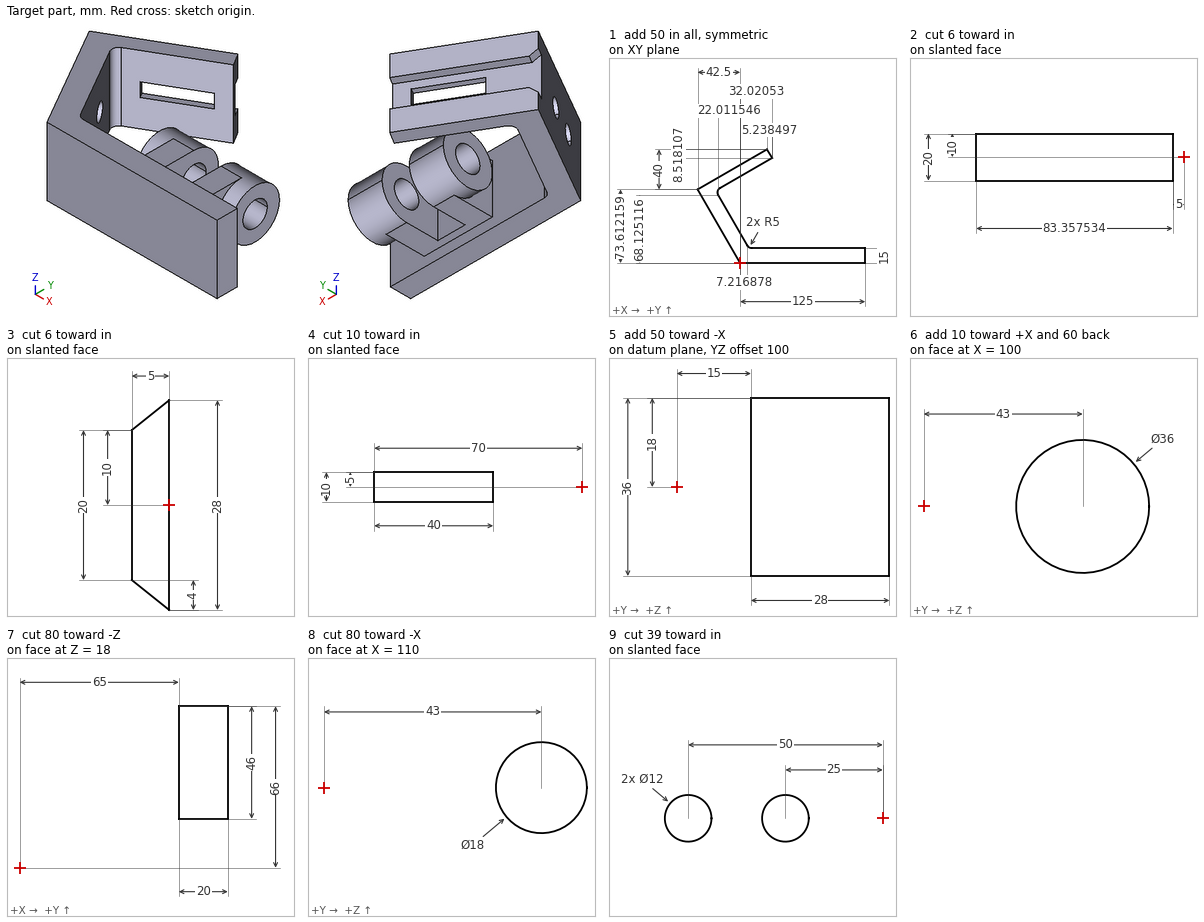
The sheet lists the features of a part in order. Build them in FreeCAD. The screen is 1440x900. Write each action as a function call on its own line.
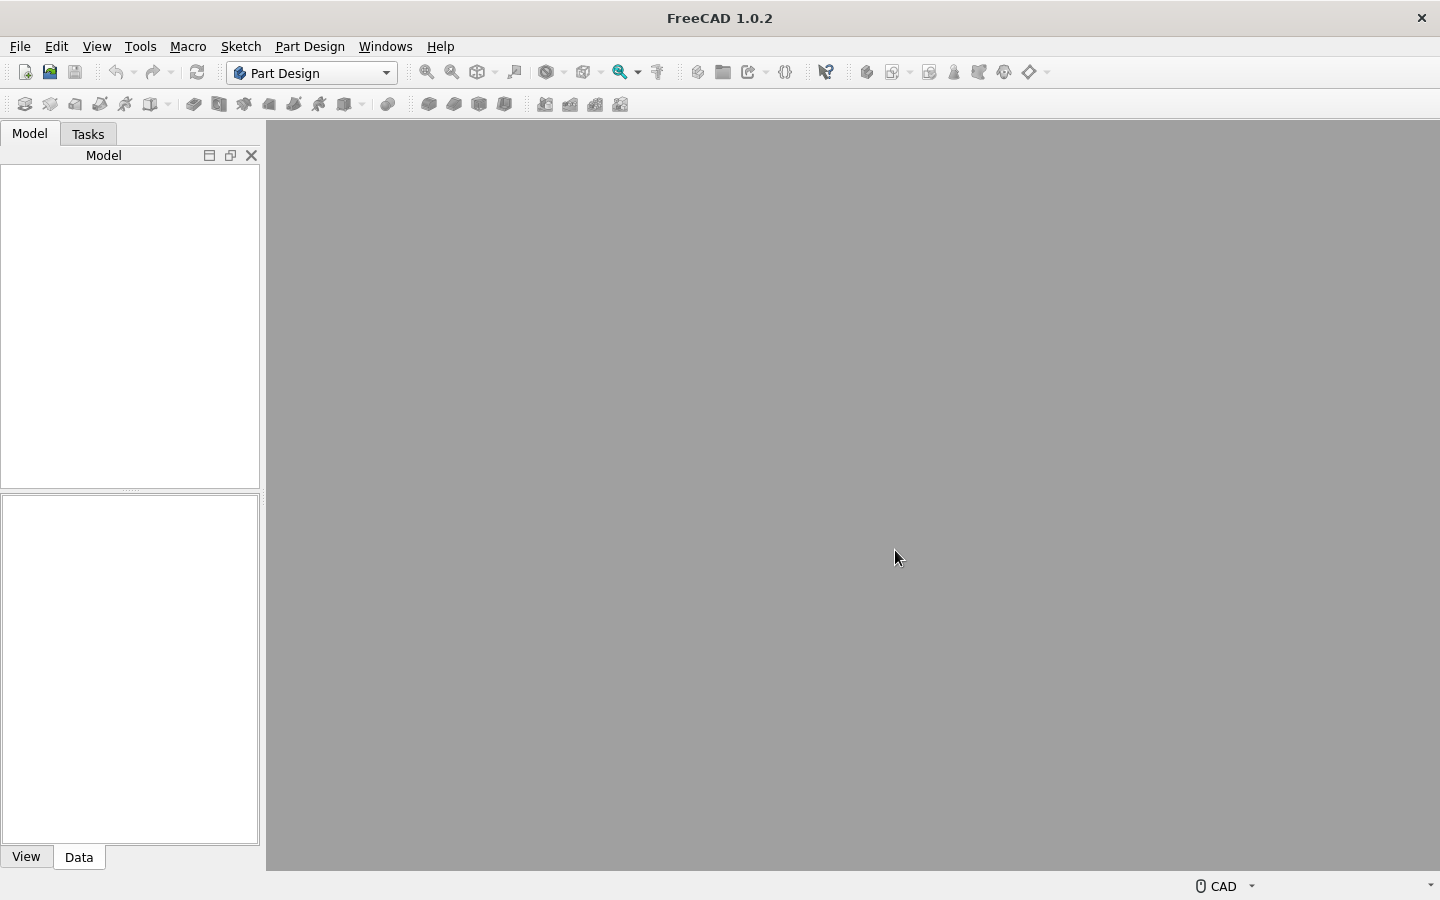
click(25, 72)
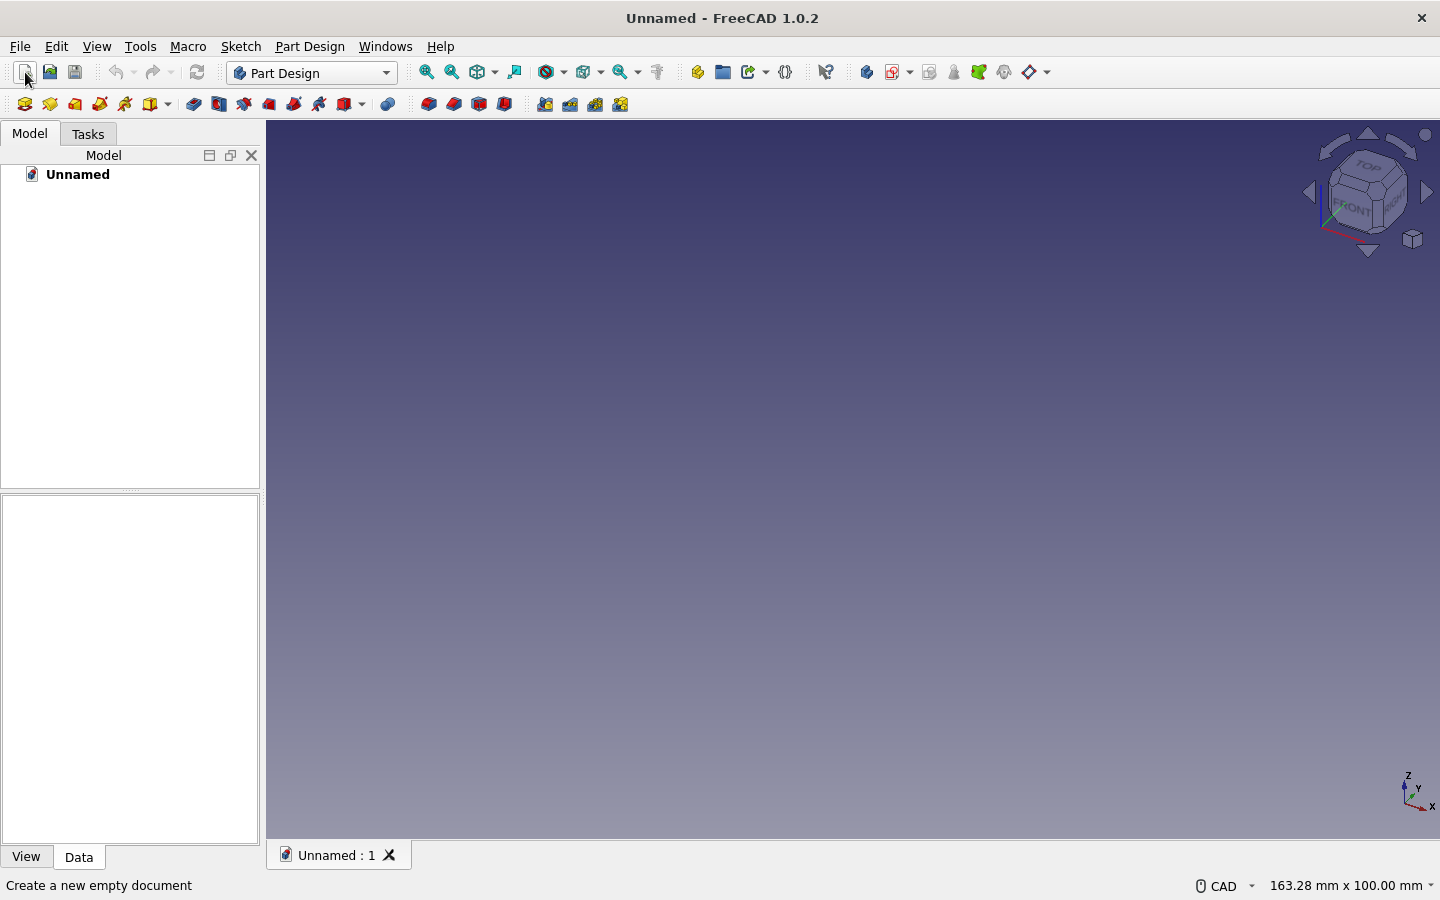
click(892, 72)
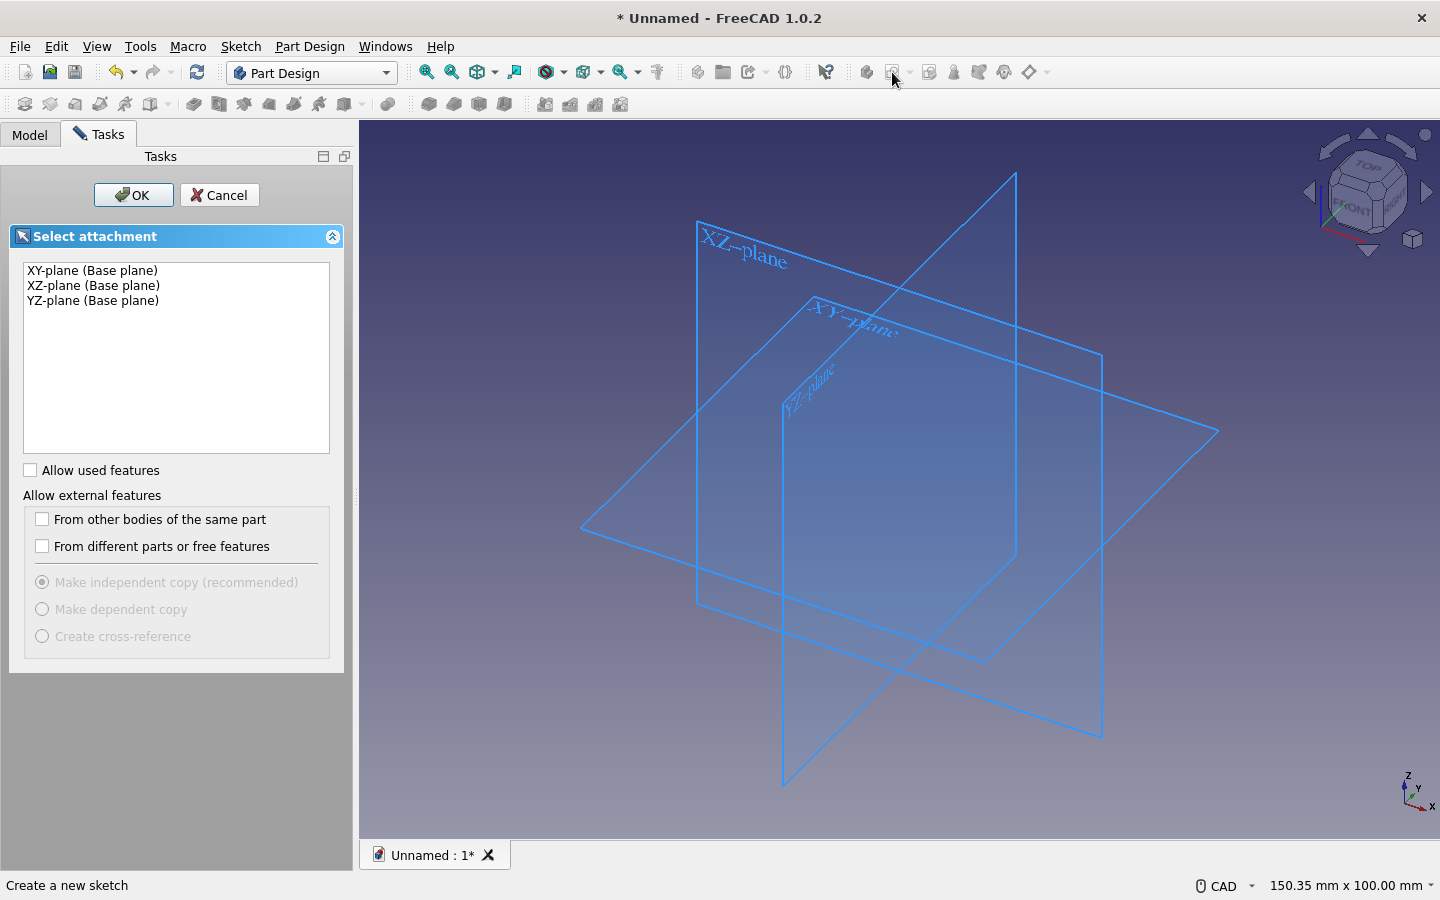
click(84, 270)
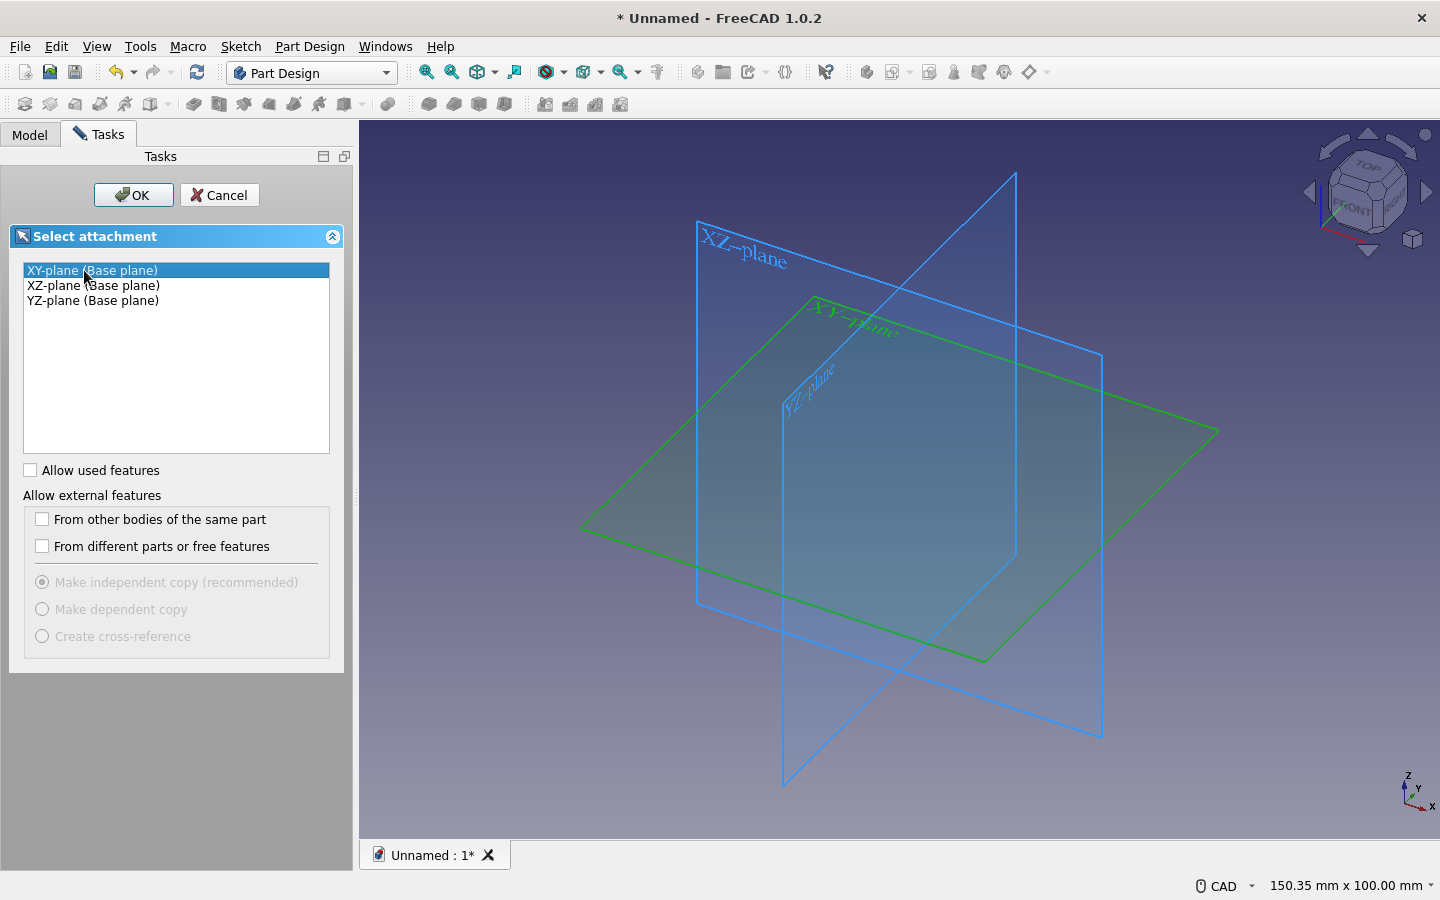
click(134, 195)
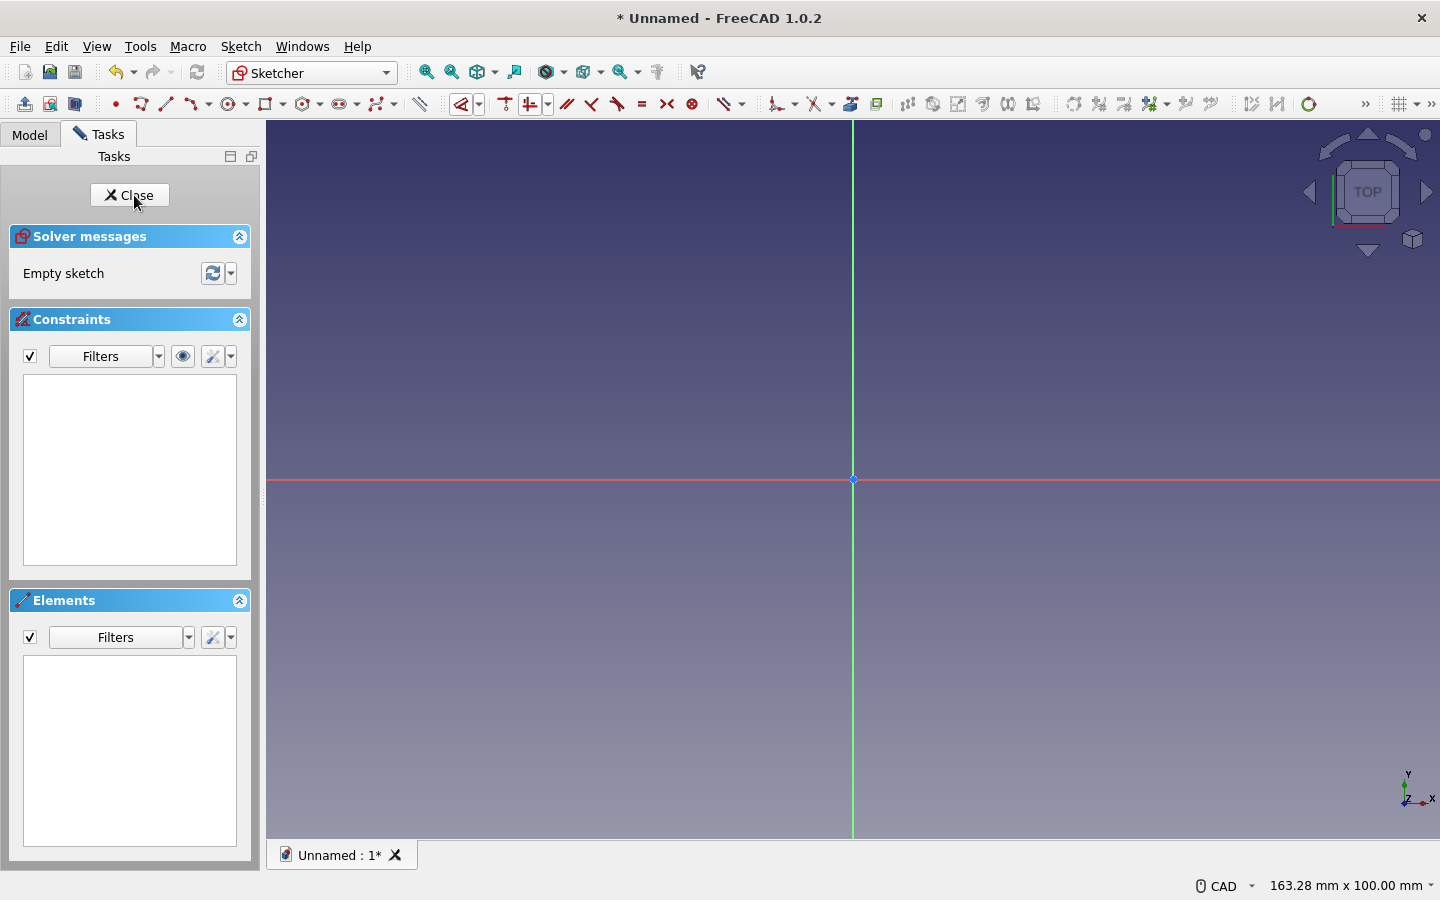
scroll(340, 811, down, 3)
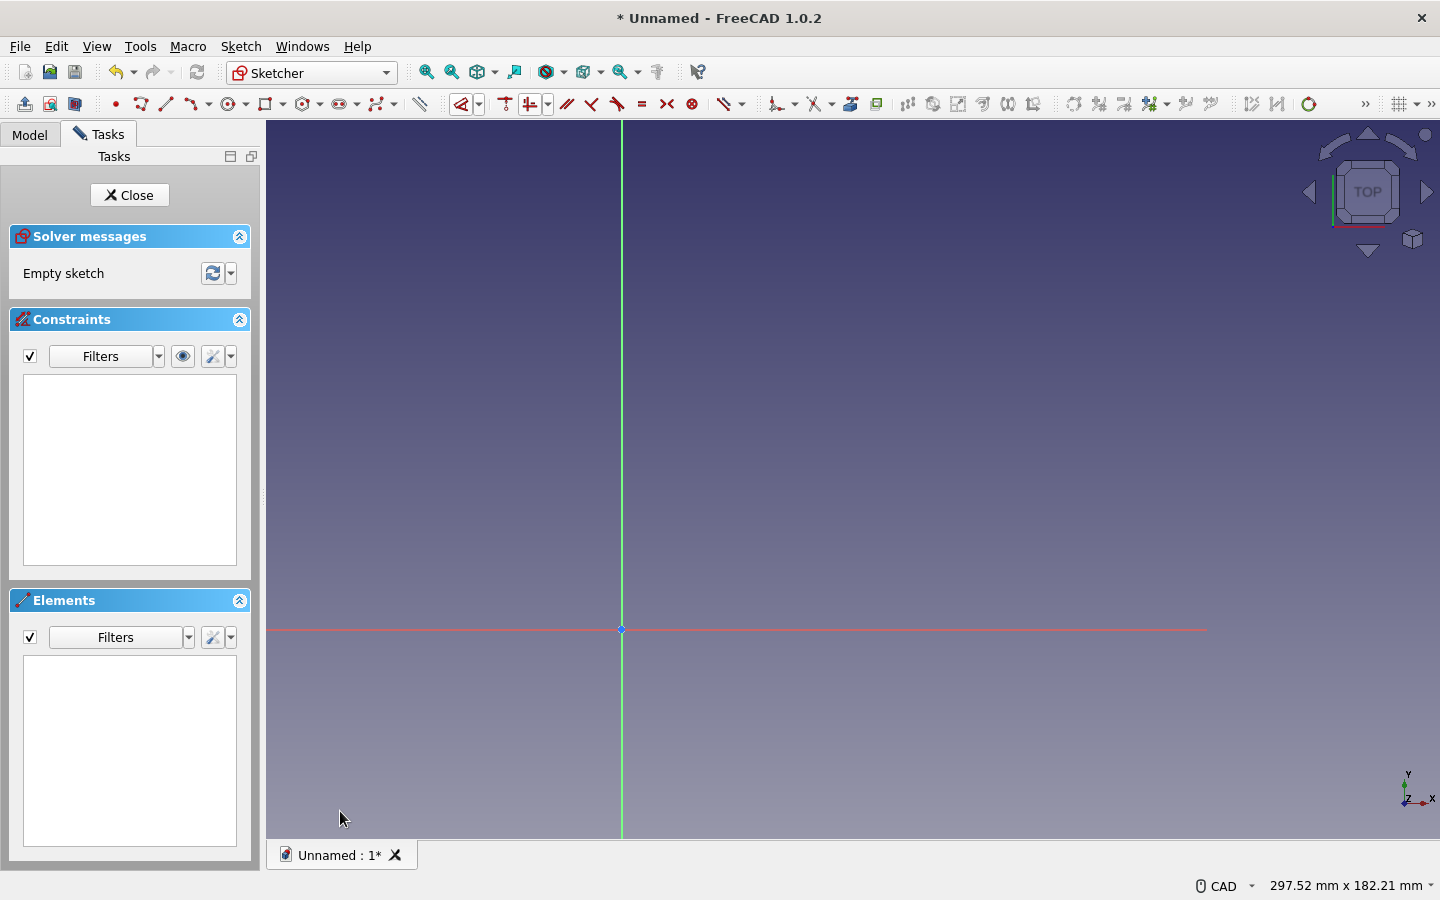
key(g)
key(l)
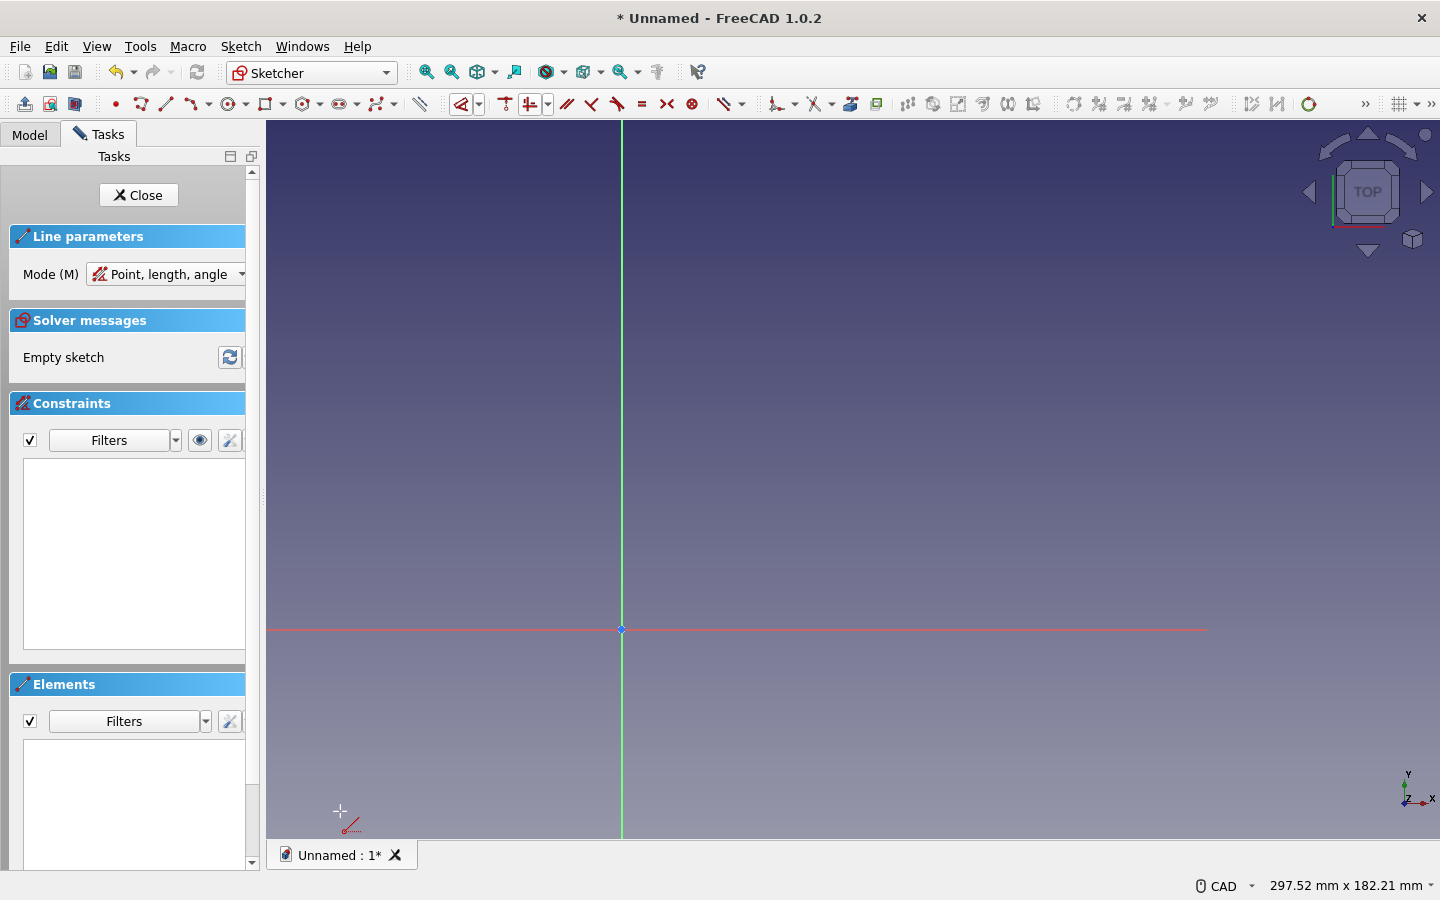
click(650, 560)
click(535, 361)